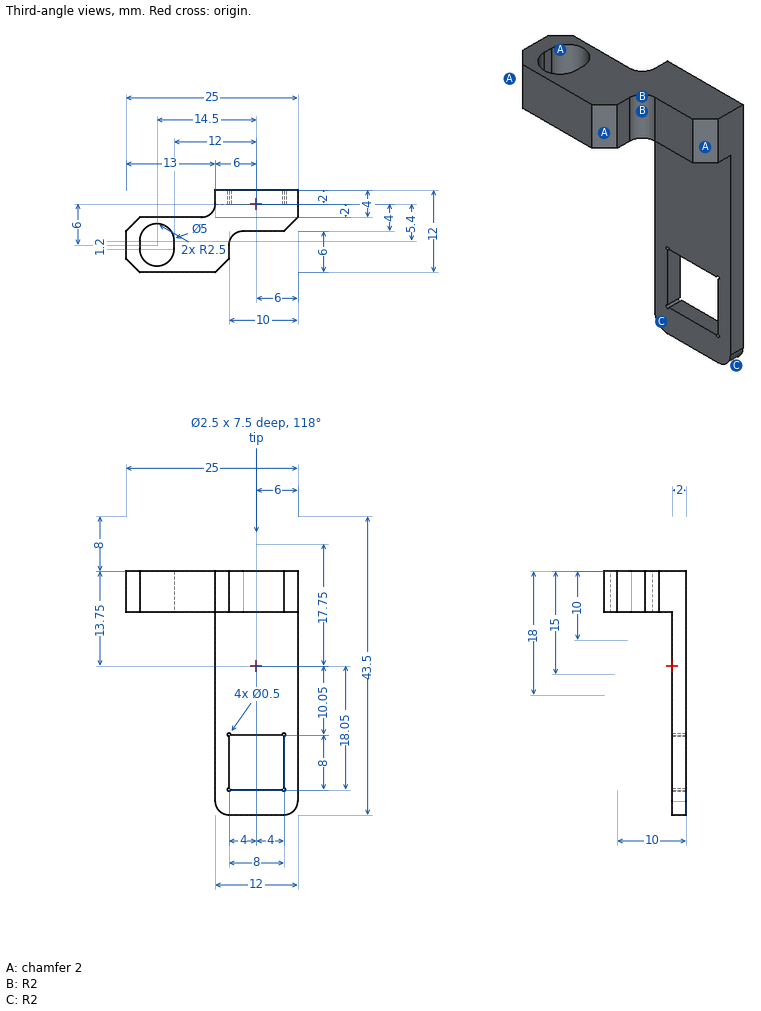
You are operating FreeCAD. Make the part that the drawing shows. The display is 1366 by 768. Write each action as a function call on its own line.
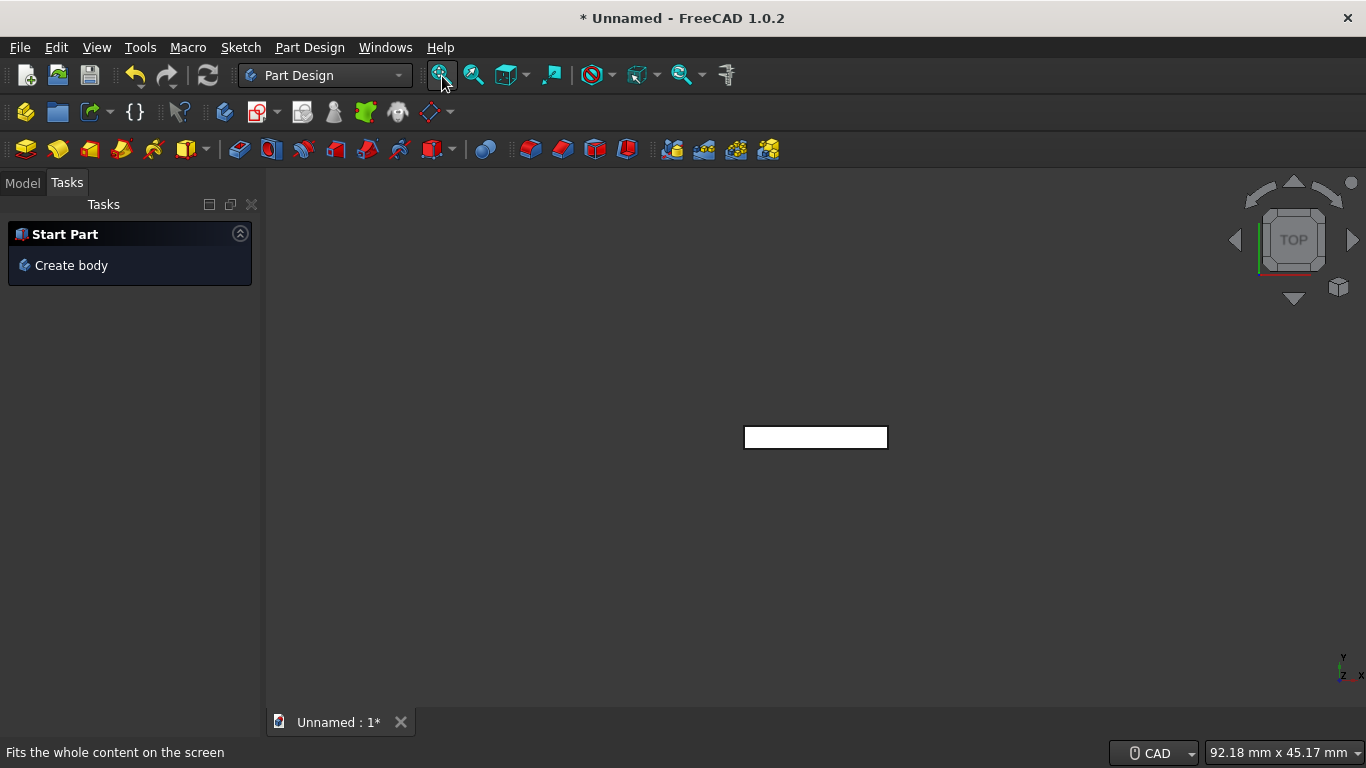
click(857, 436)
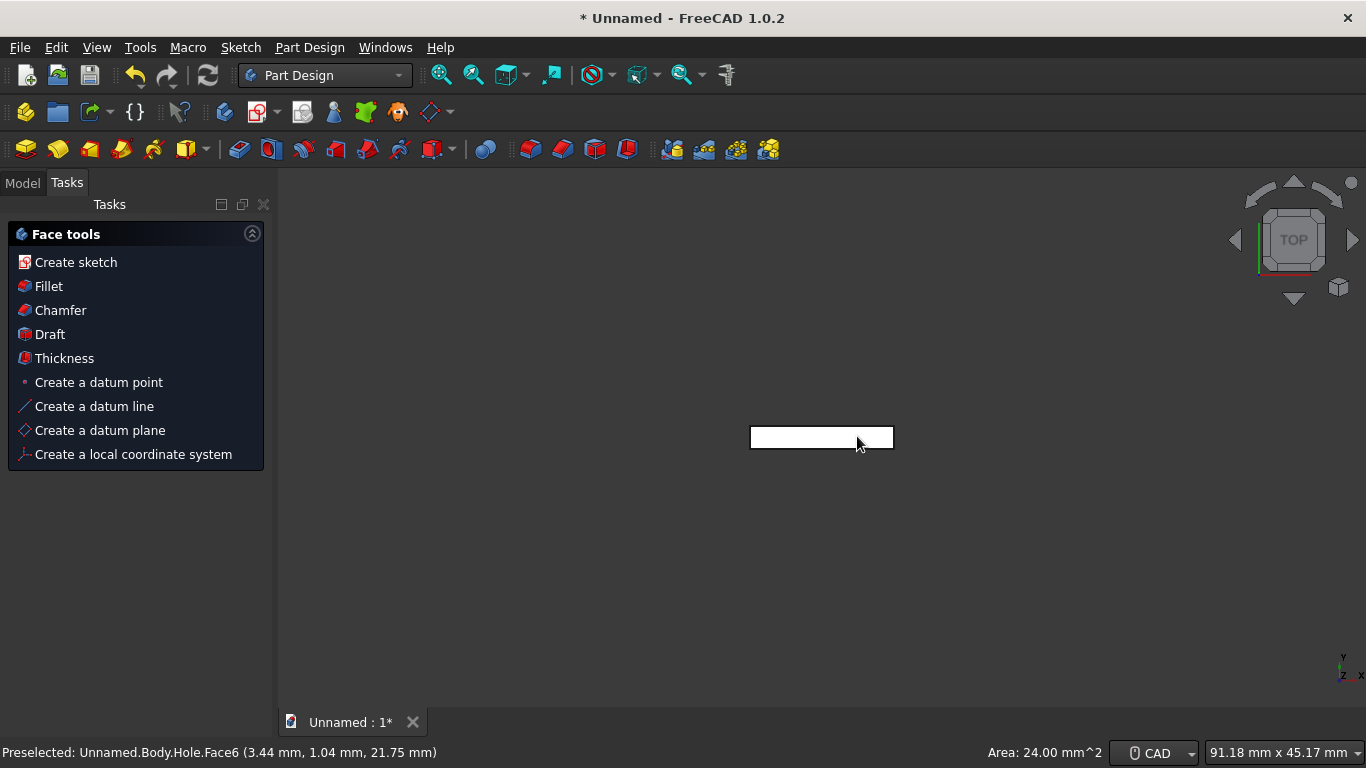
click(258, 112)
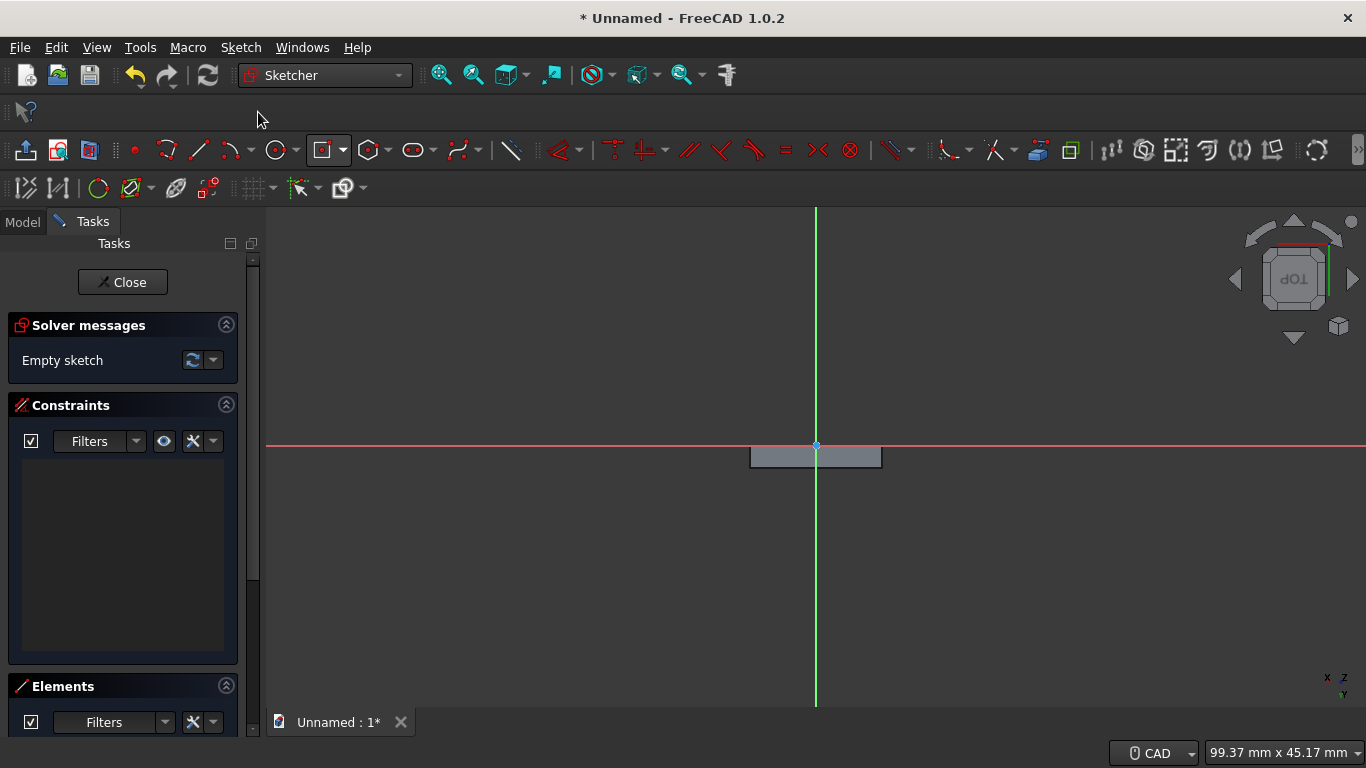
scroll(1003, 356, up, 4)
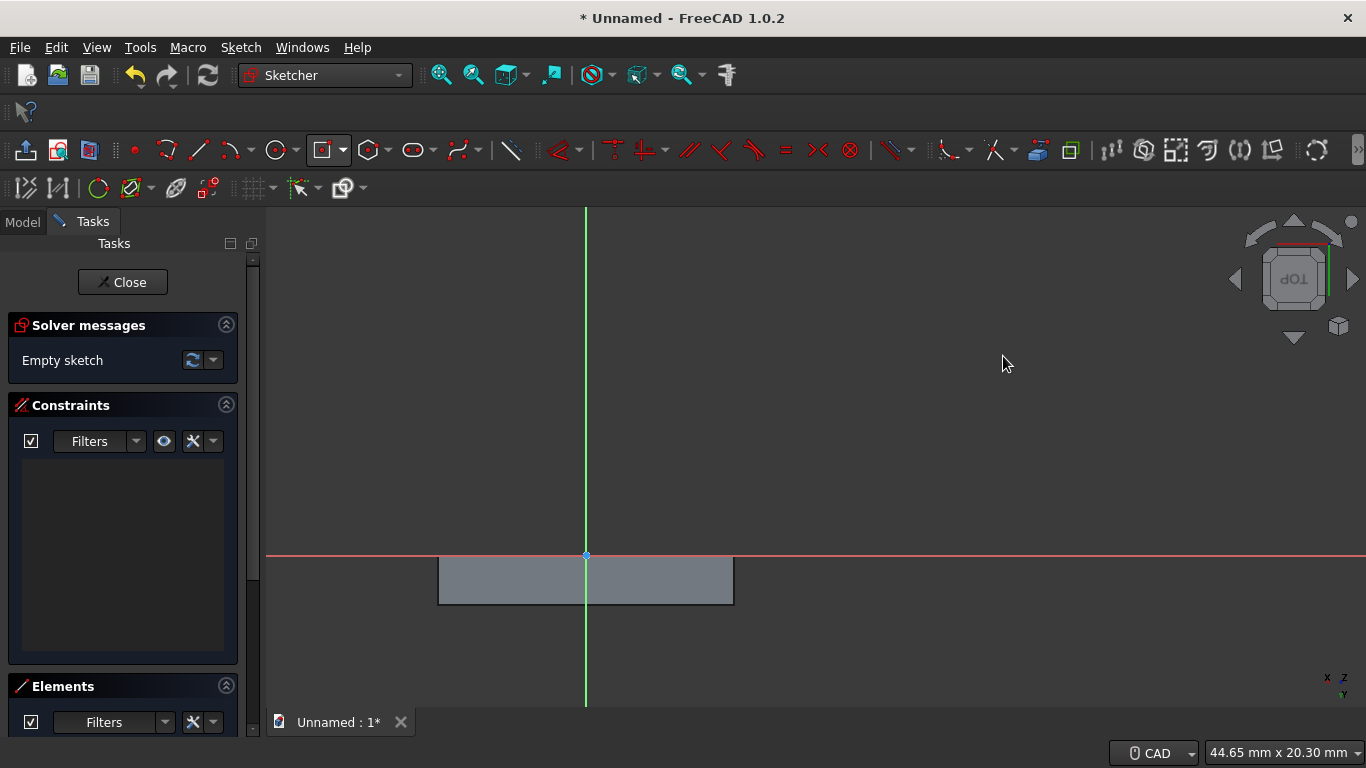
click(346, 150)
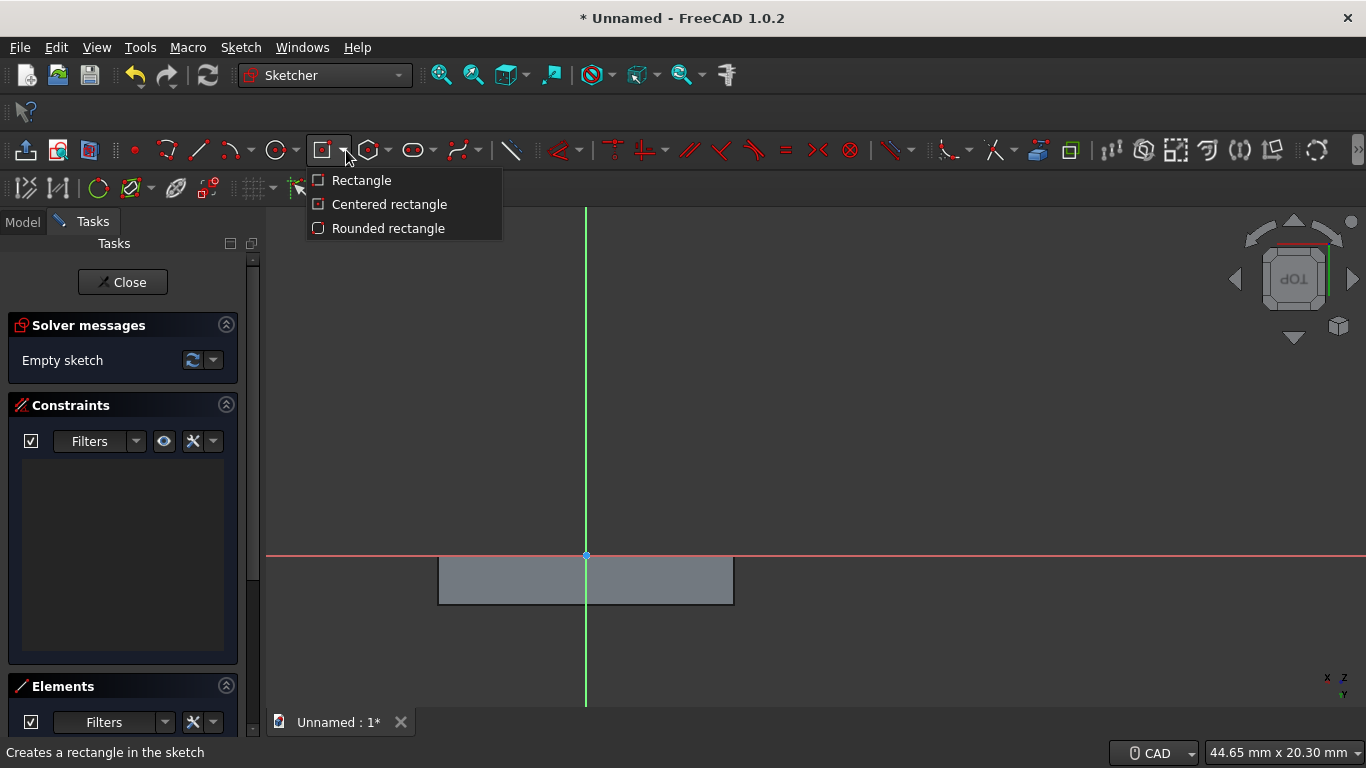
click(404, 180)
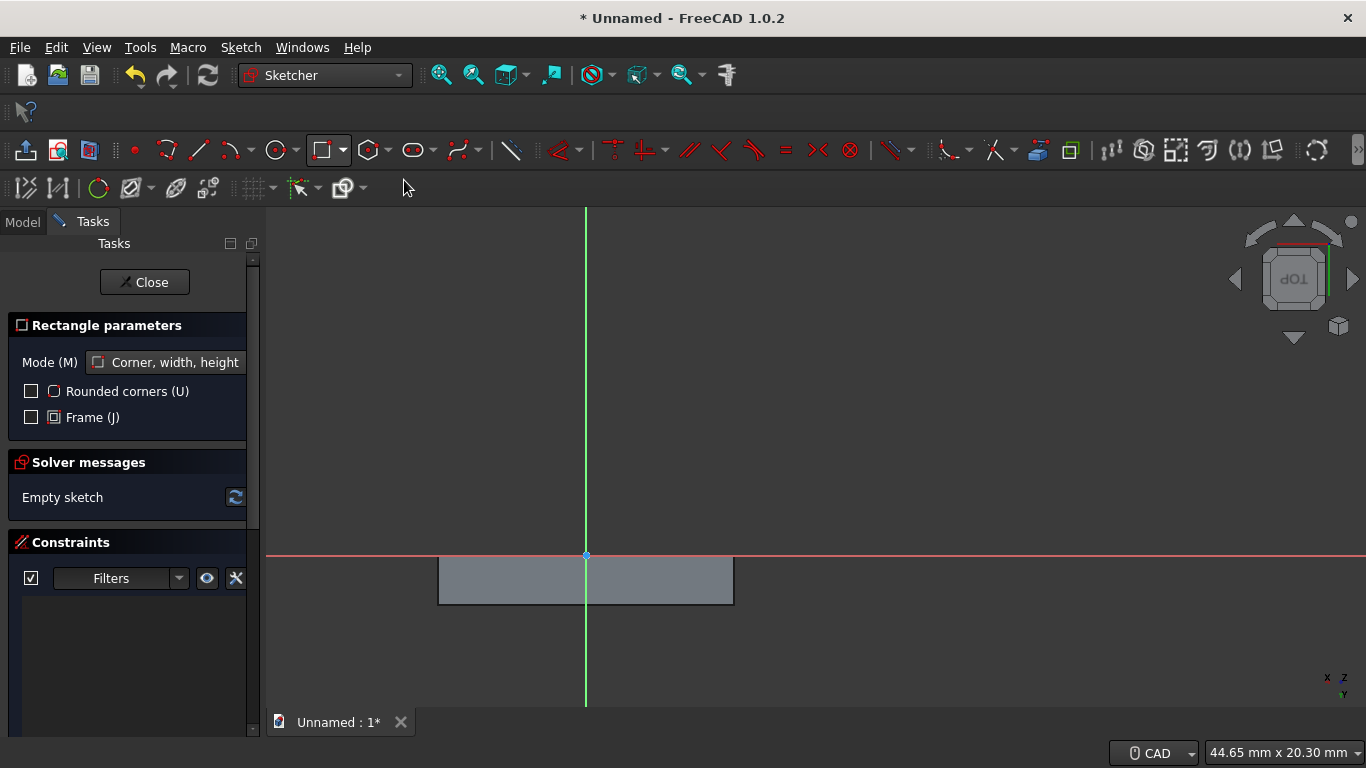
click(438, 309)
click(1054, 605)
key(Escape)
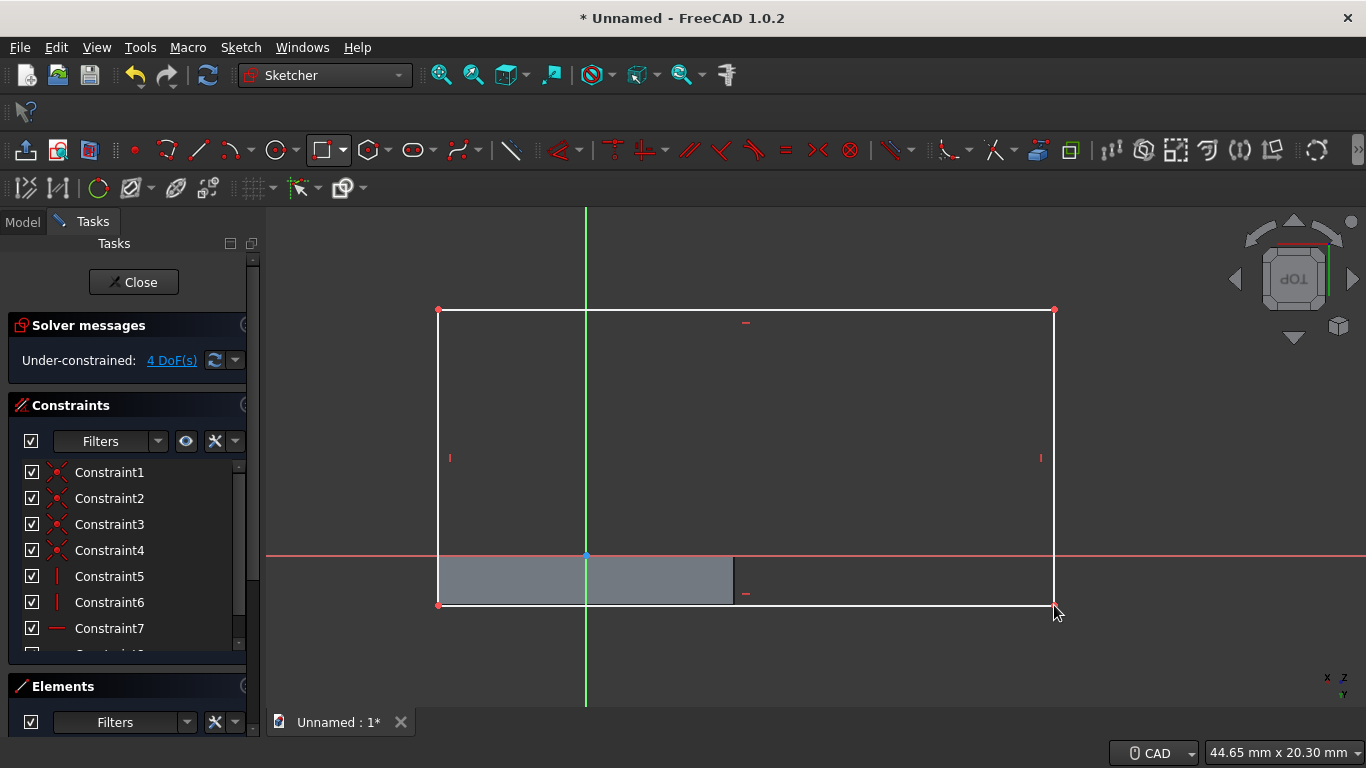
click(558, 150)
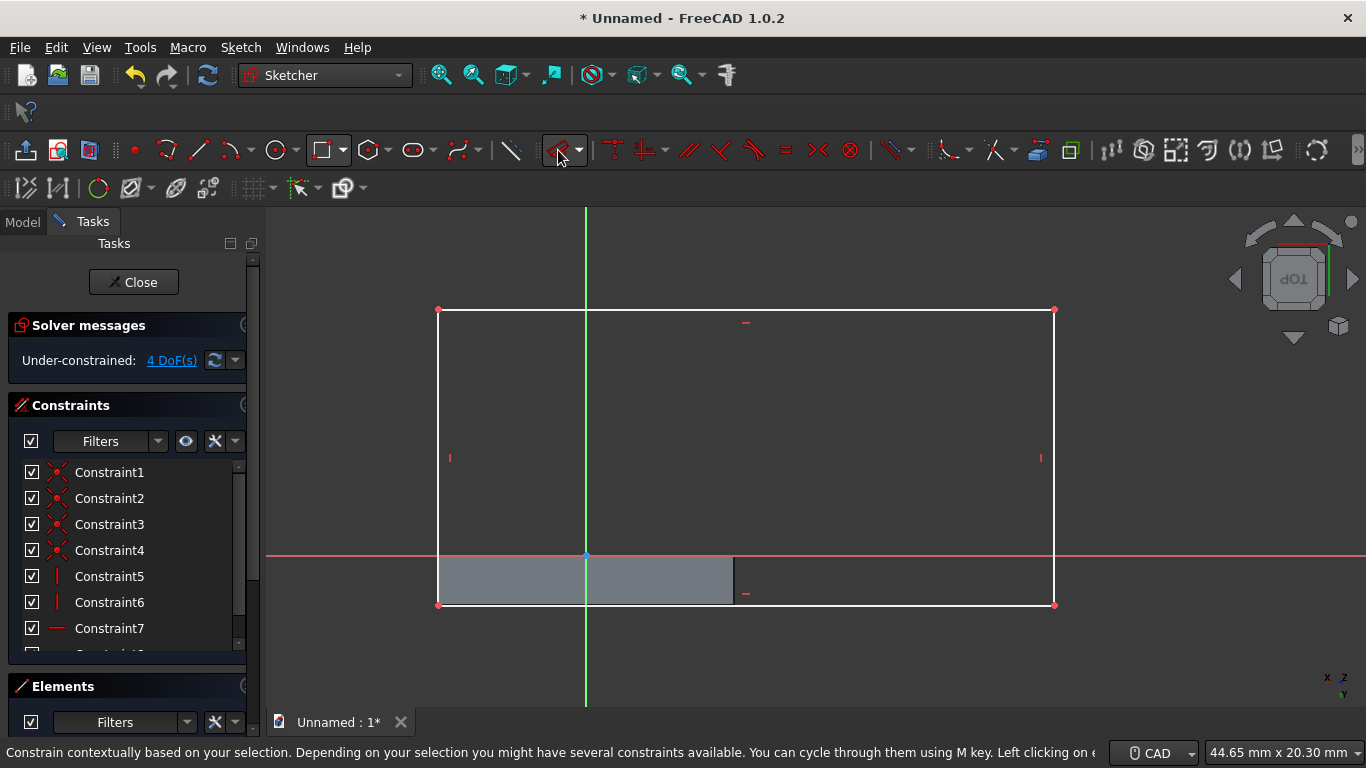
click(438, 399)
click(404, 458)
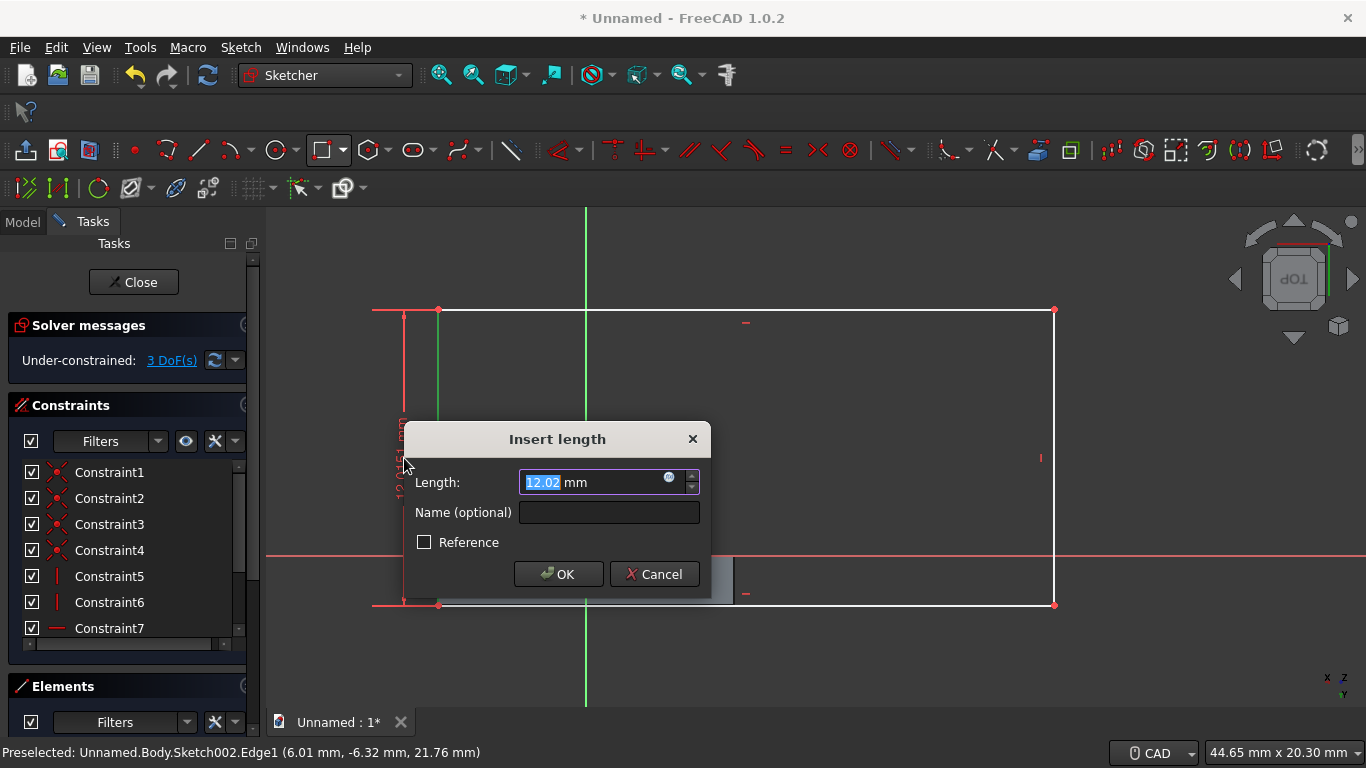
text(12)
key(Return)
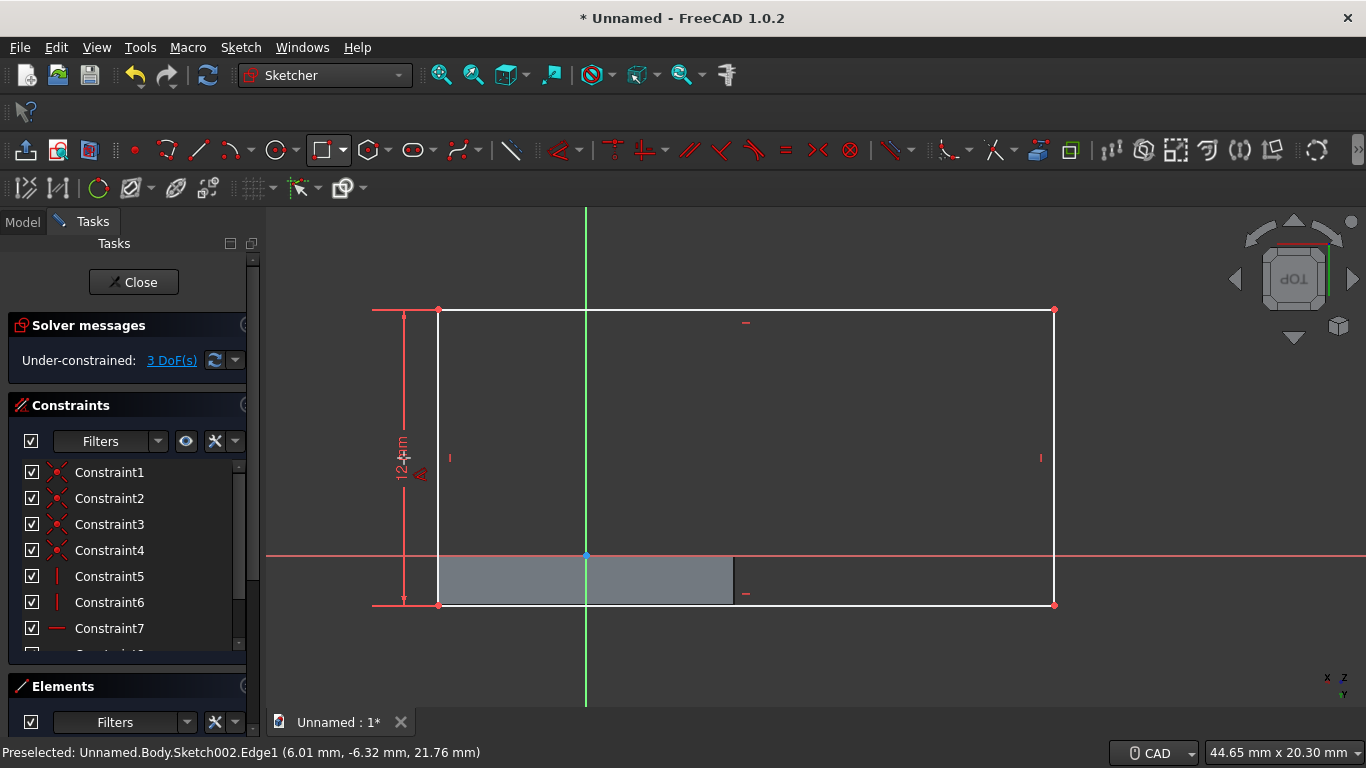
click(623, 606)
click(746, 640)